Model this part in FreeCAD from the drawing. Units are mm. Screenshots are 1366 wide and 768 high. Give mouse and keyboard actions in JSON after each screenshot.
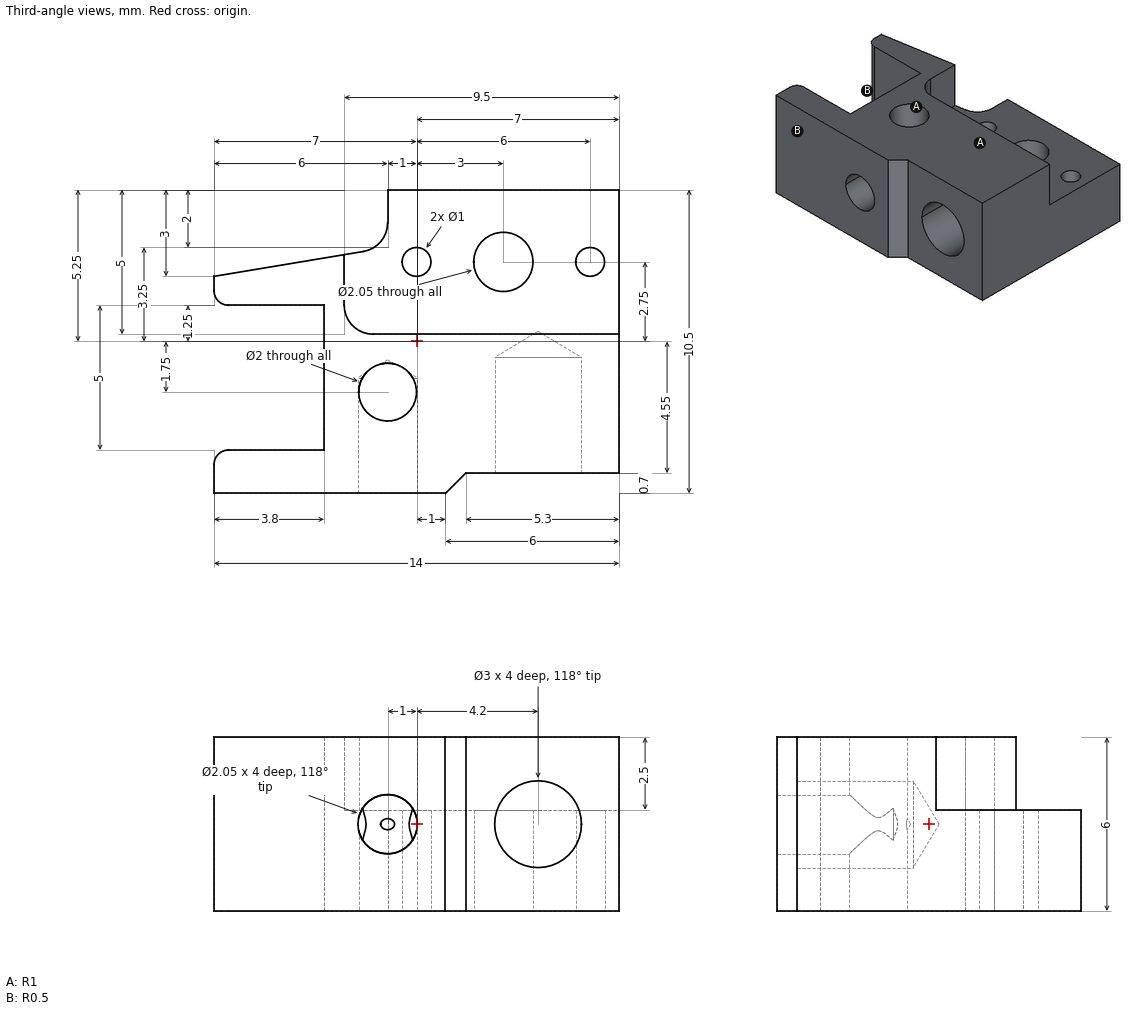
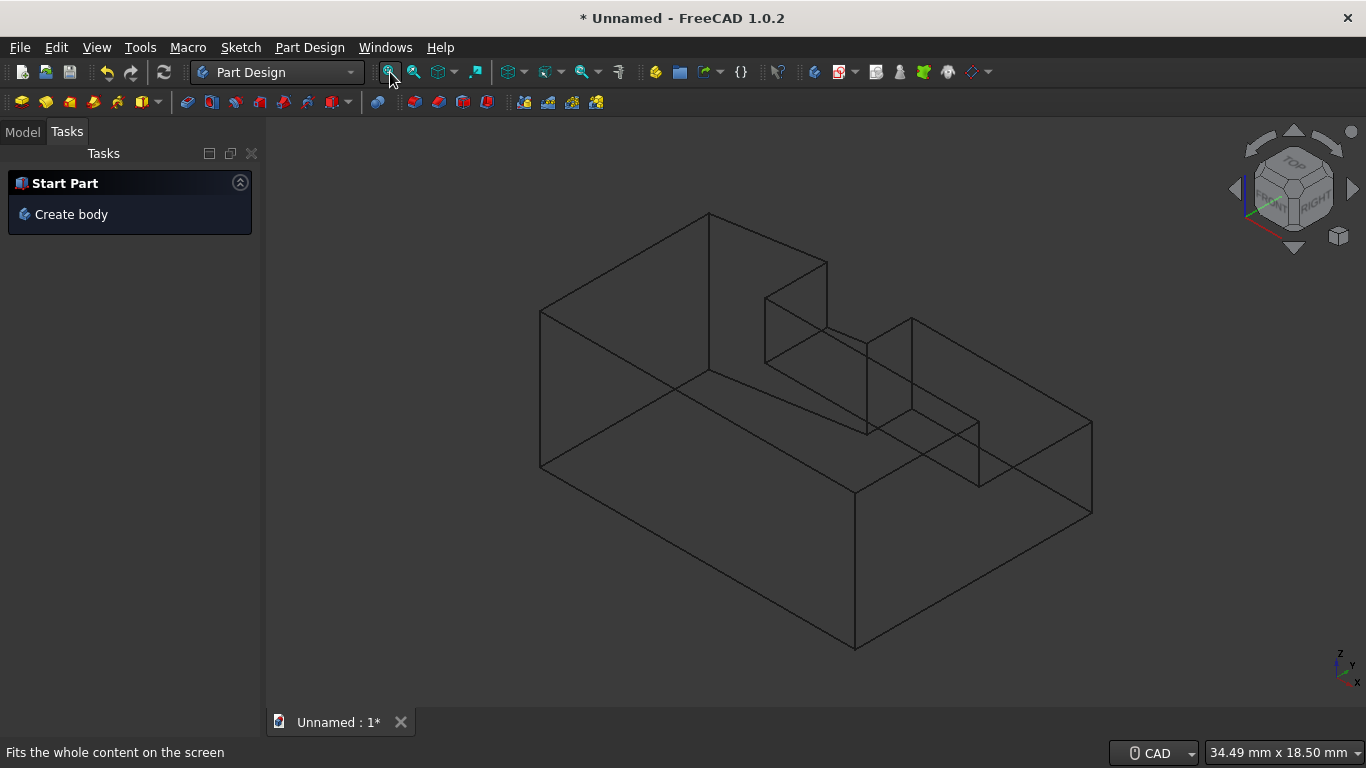
{"action": "left_click", "coordinate": [765, 330]}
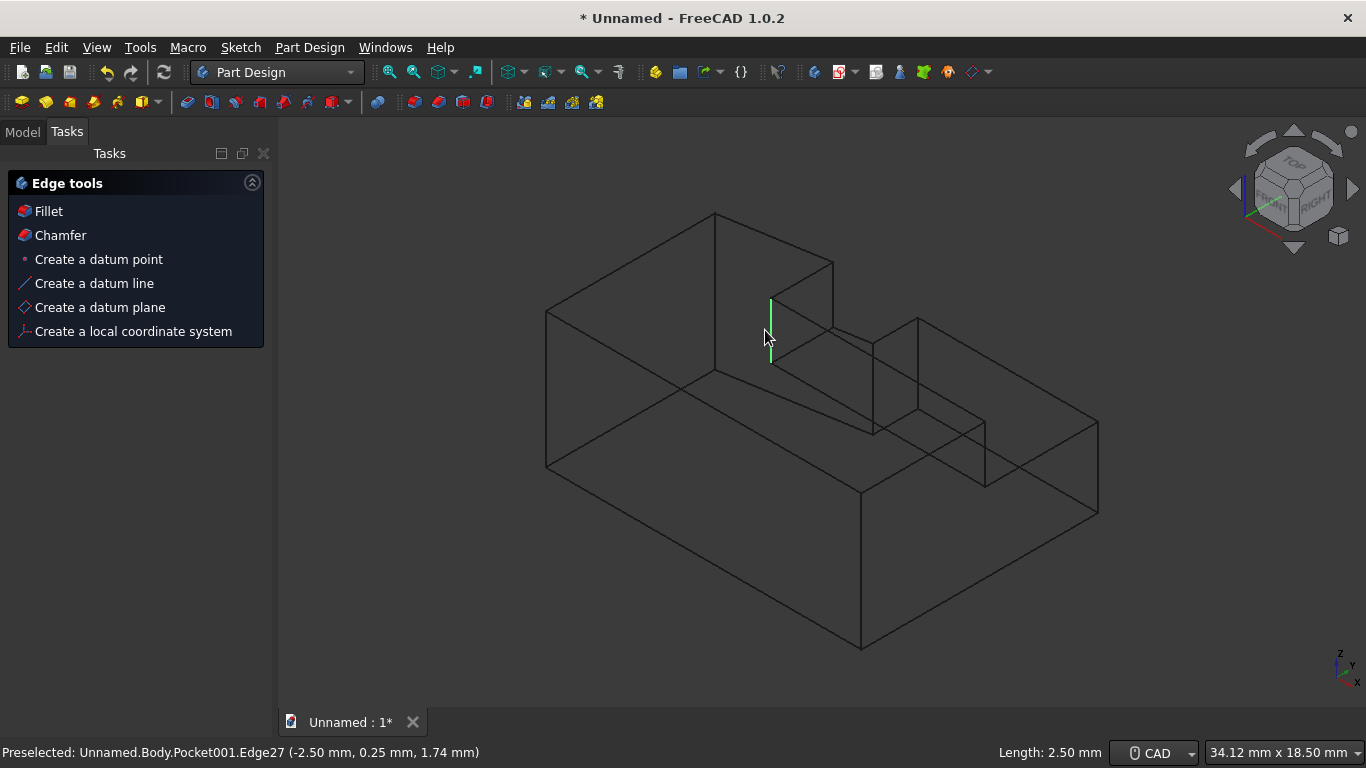
{"action": "left_click", "coordinate": [873, 388], "text": "ctrl"}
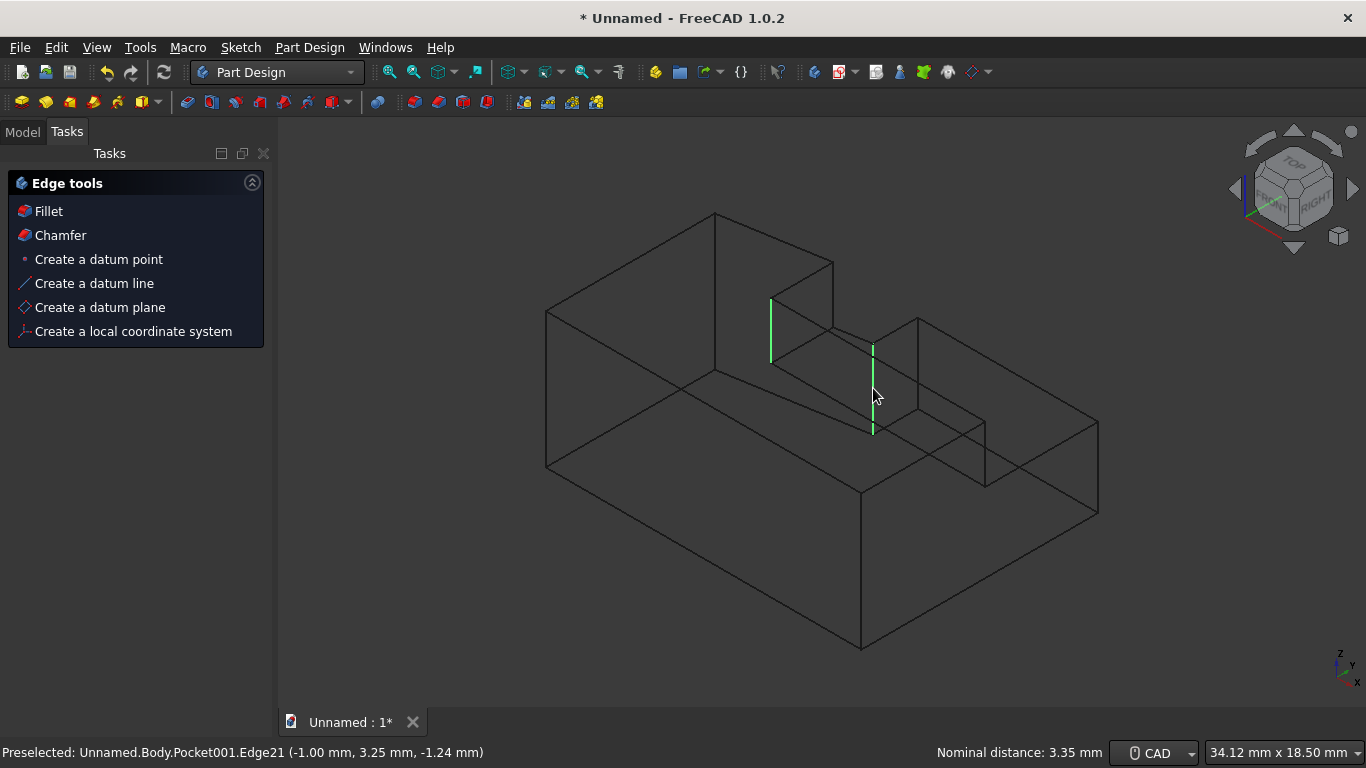
{"action": "key", "text": "v 1"}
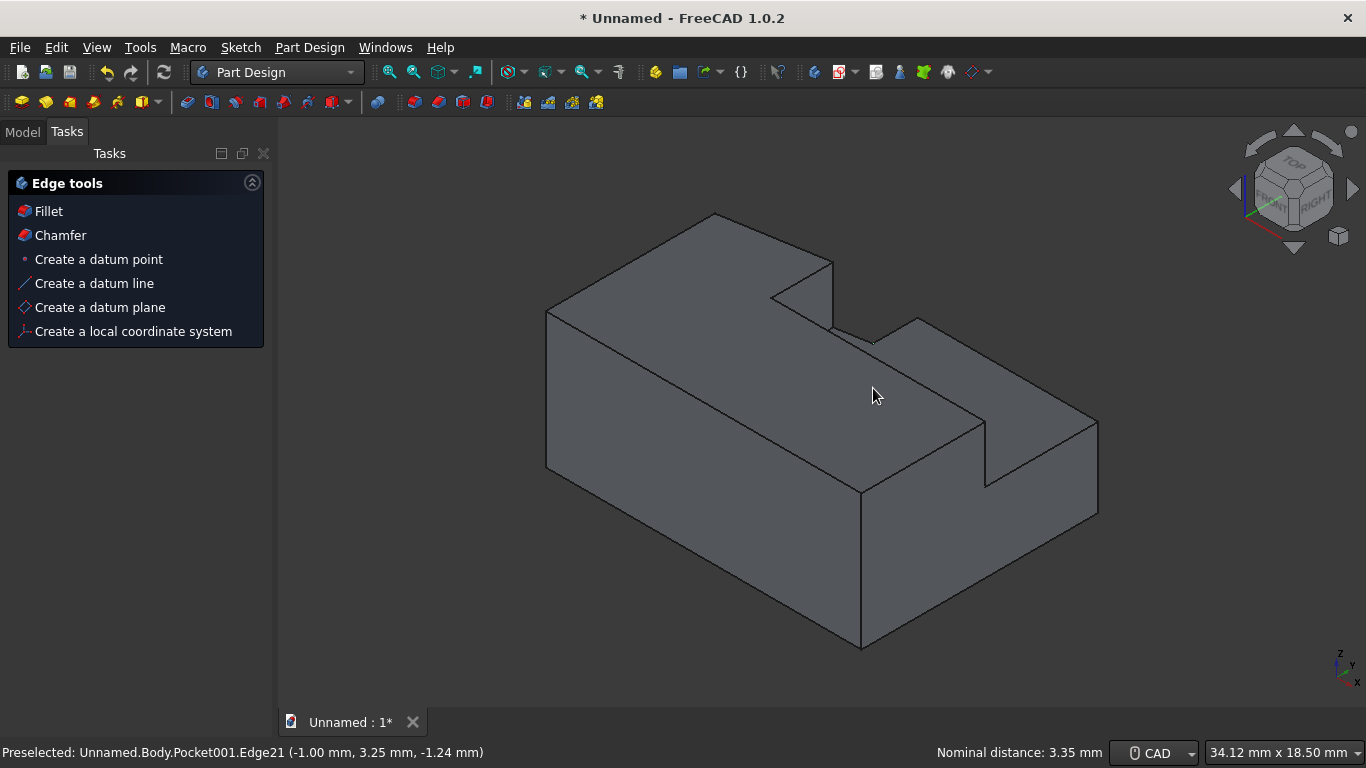
{"action": "left_click", "coordinate": [416, 102]}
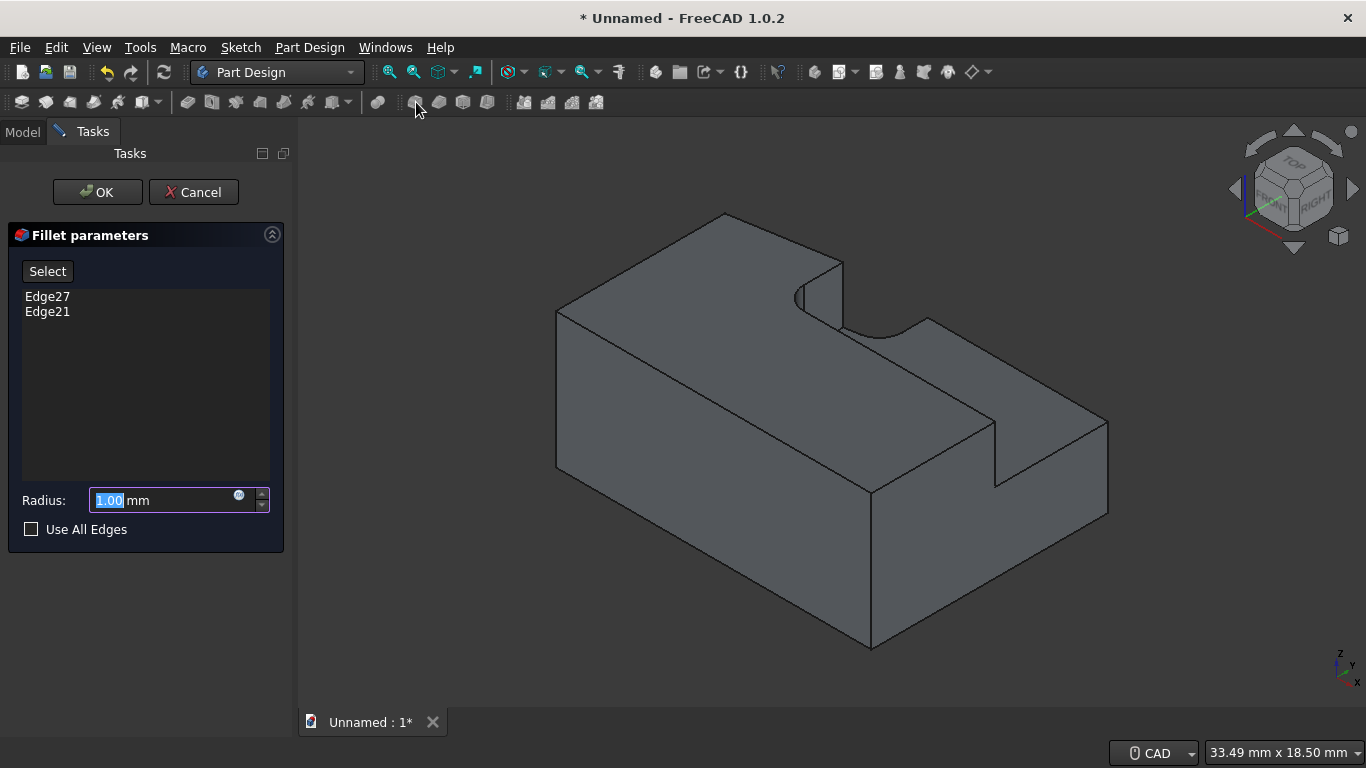
{"action": "type", "text": "1"}
{"action": "key", "text": "Tab"}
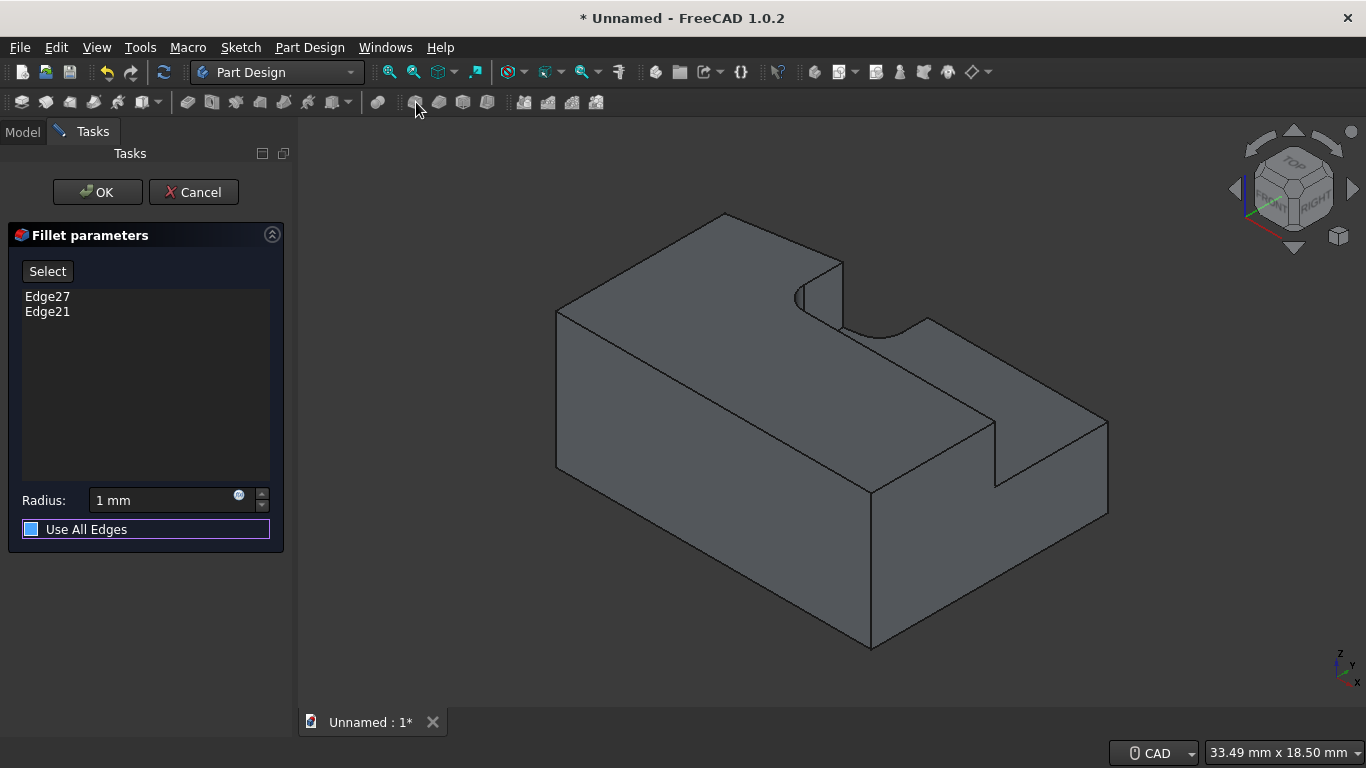
{"action": "left_click", "coordinate": [98, 192]}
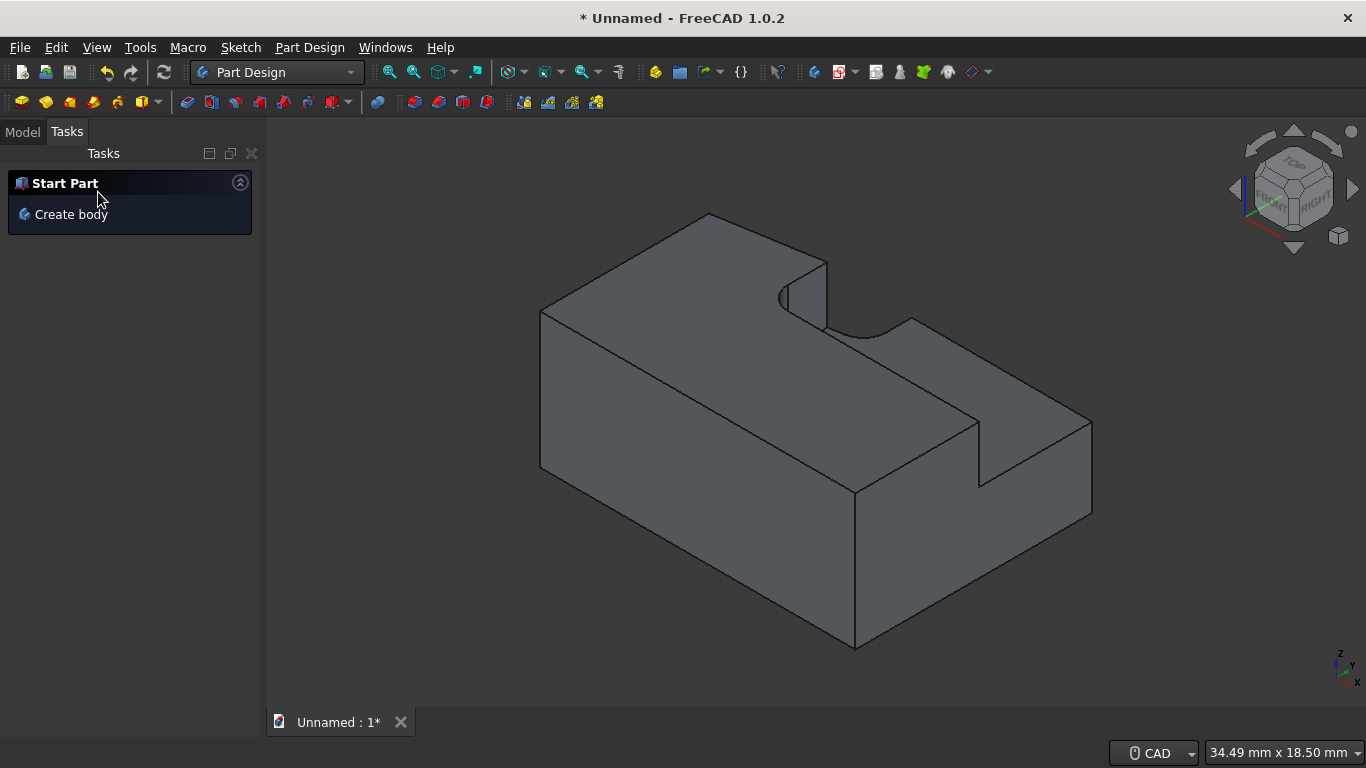
{"action": "left_click", "coordinate": [674, 311]}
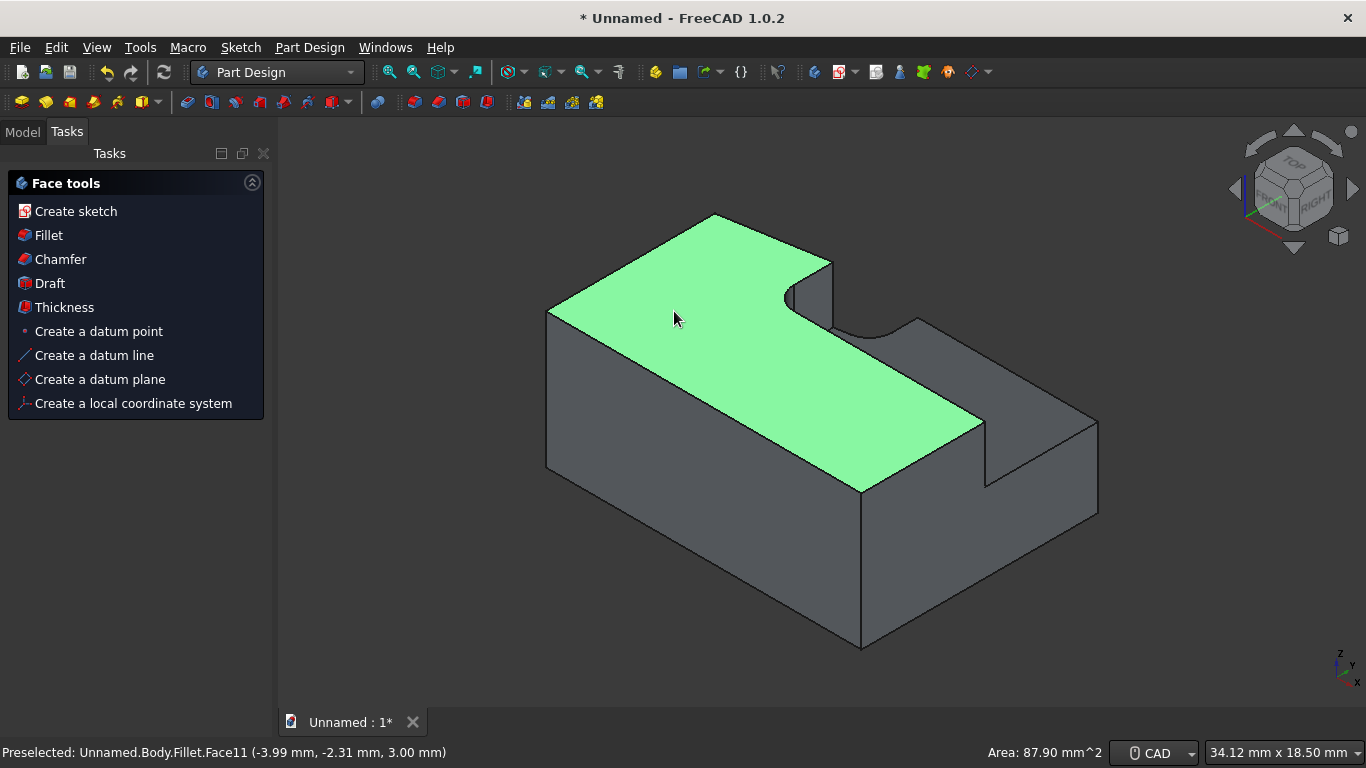
{"action": "left_click", "coordinate": [840, 72]}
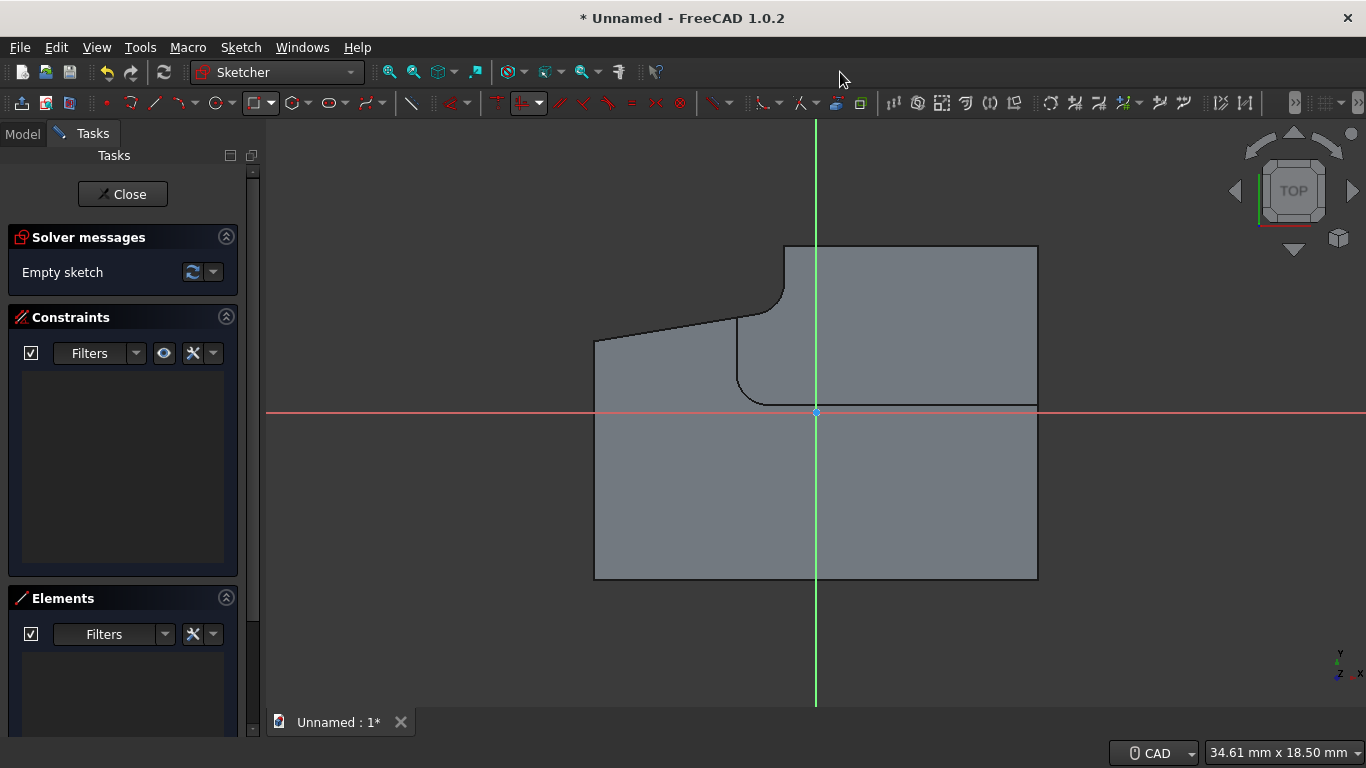
{"action": "scroll", "coordinate": [670, 485], "scroll_direction": "up", "scroll_amount": 4}